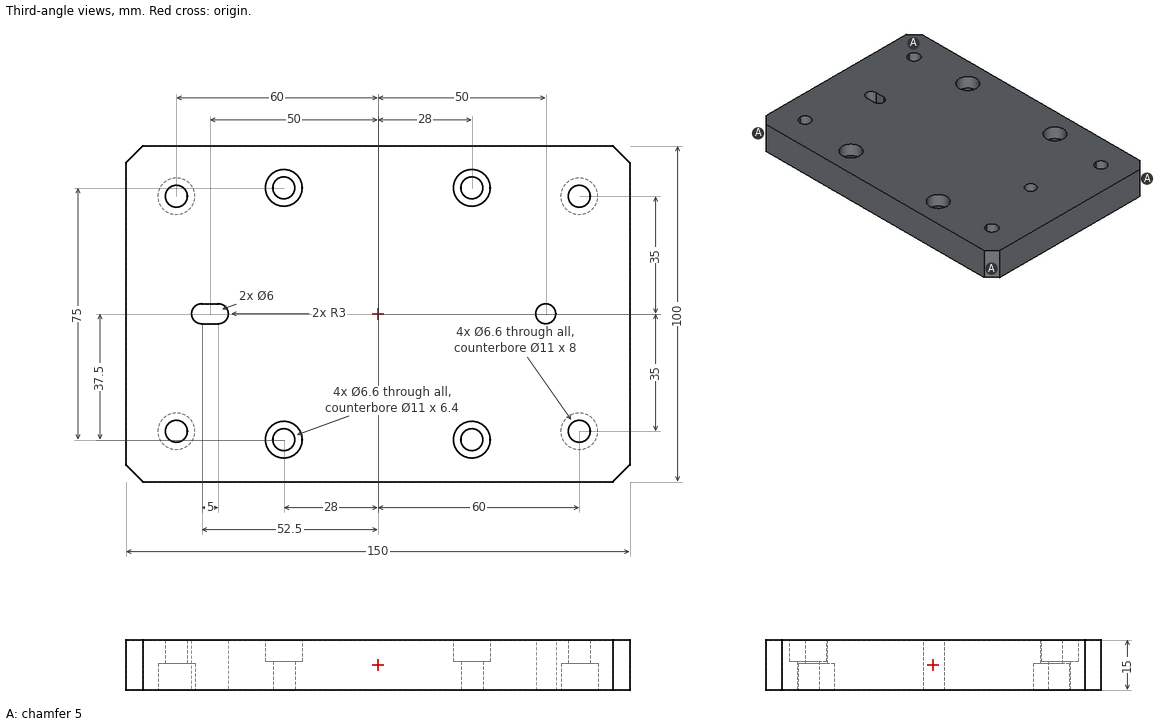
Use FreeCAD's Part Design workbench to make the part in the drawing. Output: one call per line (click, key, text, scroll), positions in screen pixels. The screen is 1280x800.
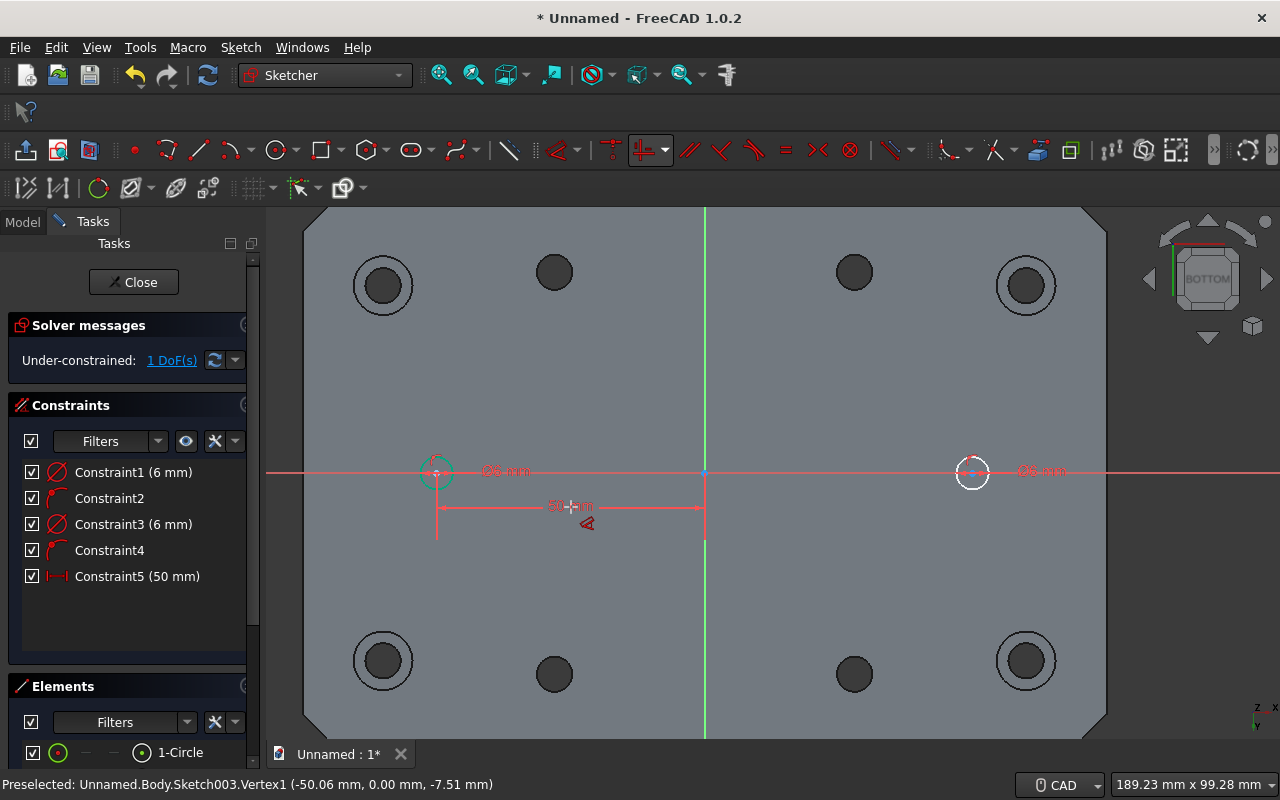
click(973, 473)
click(839, 507)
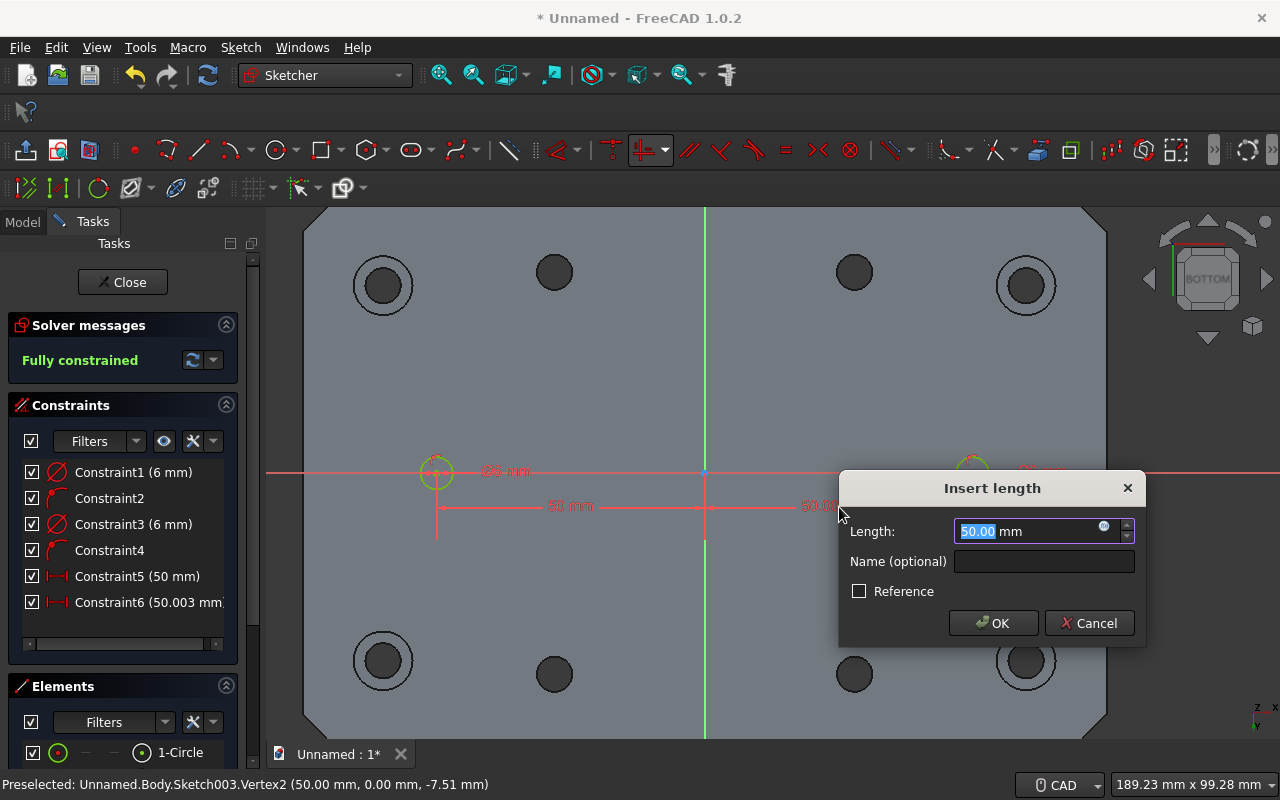
text(50)
key(Return)
key(Escape)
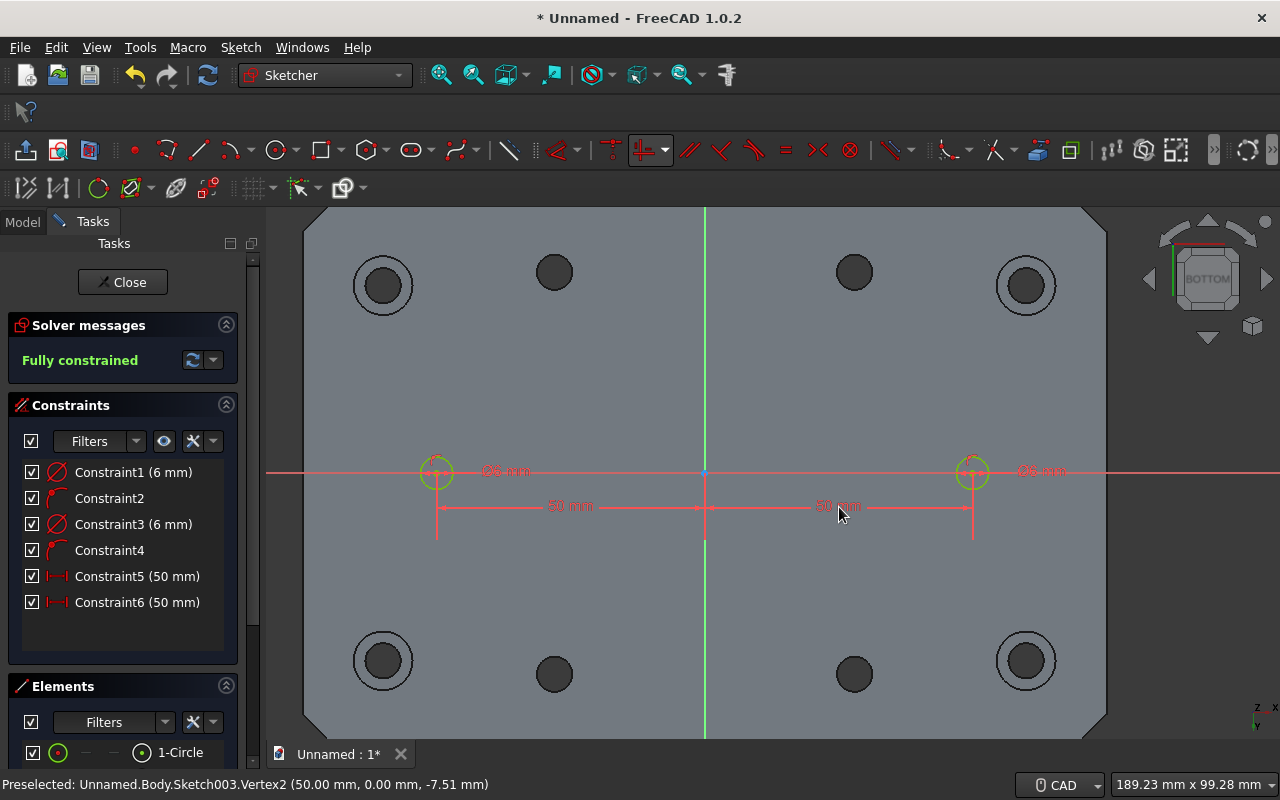
click(123, 282)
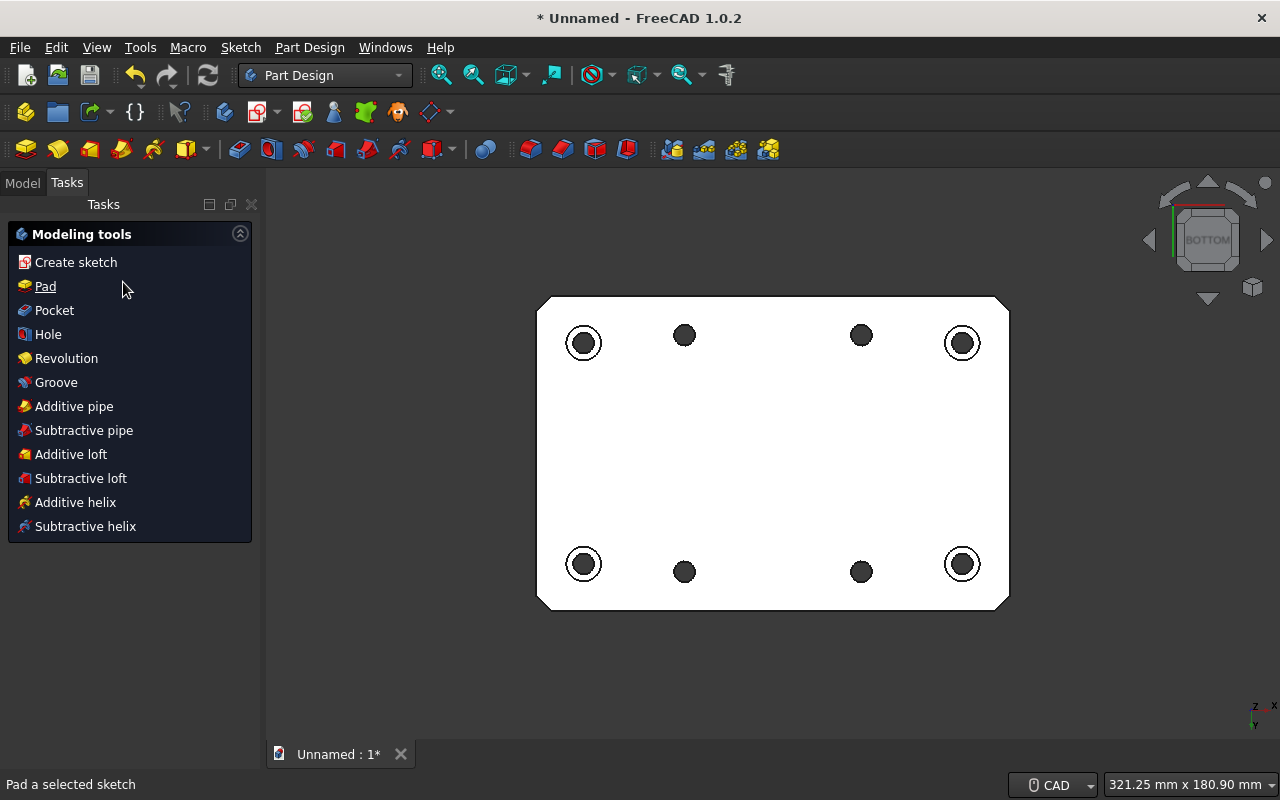
click(240, 150)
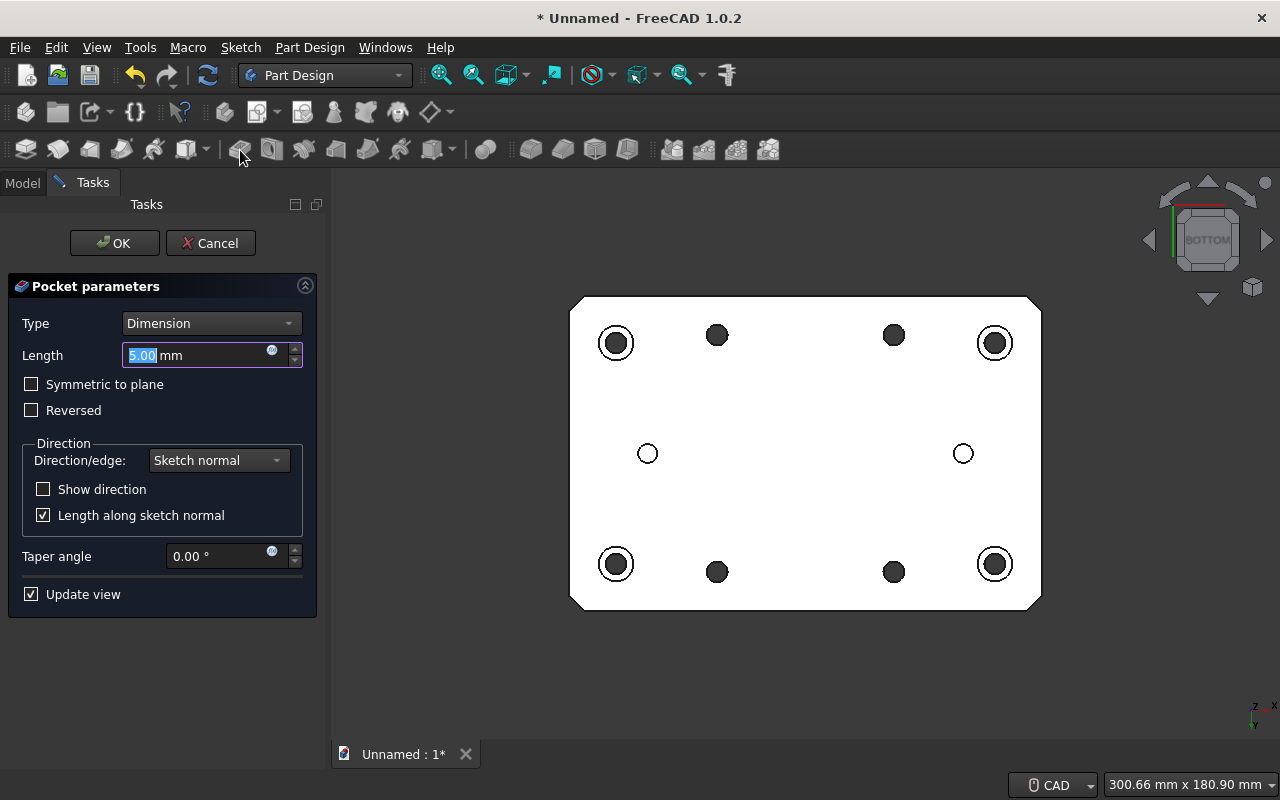
click(212, 324)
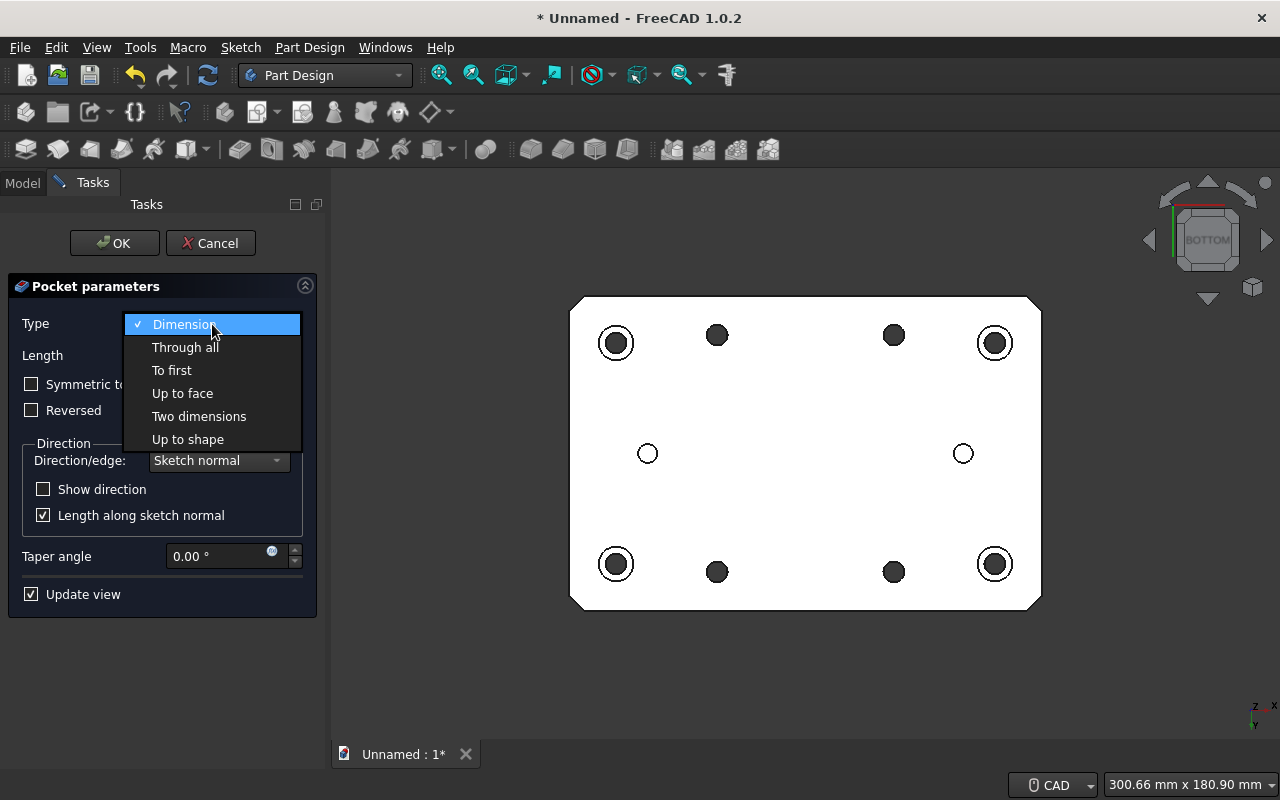
click(212, 348)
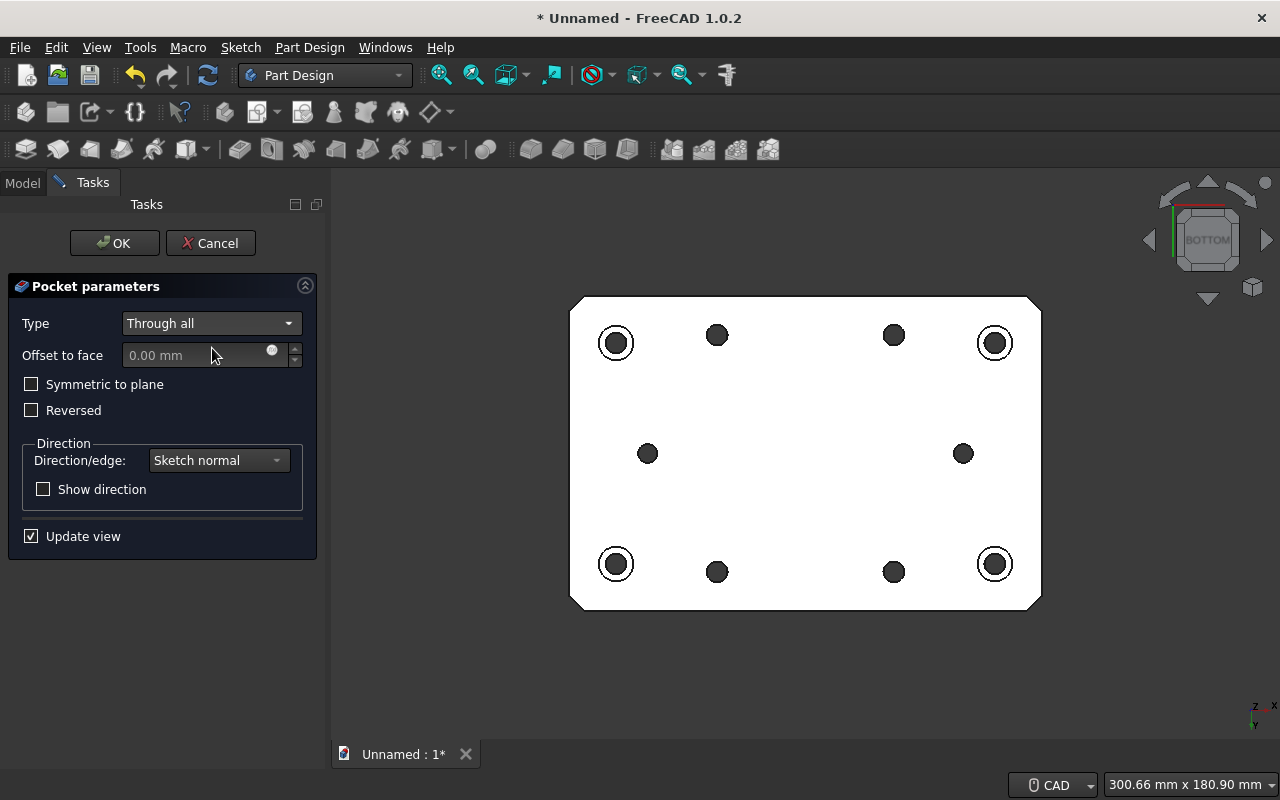
click(115, 243)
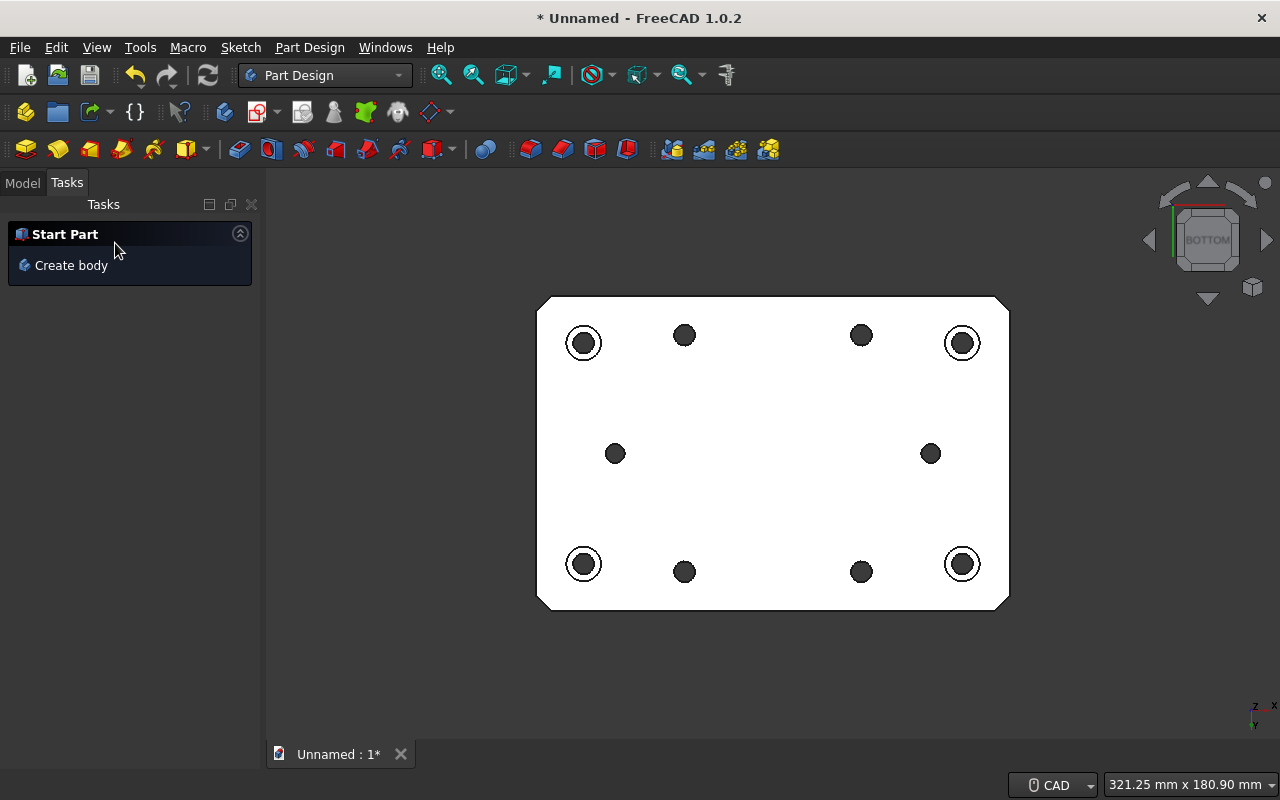
click(773, 453)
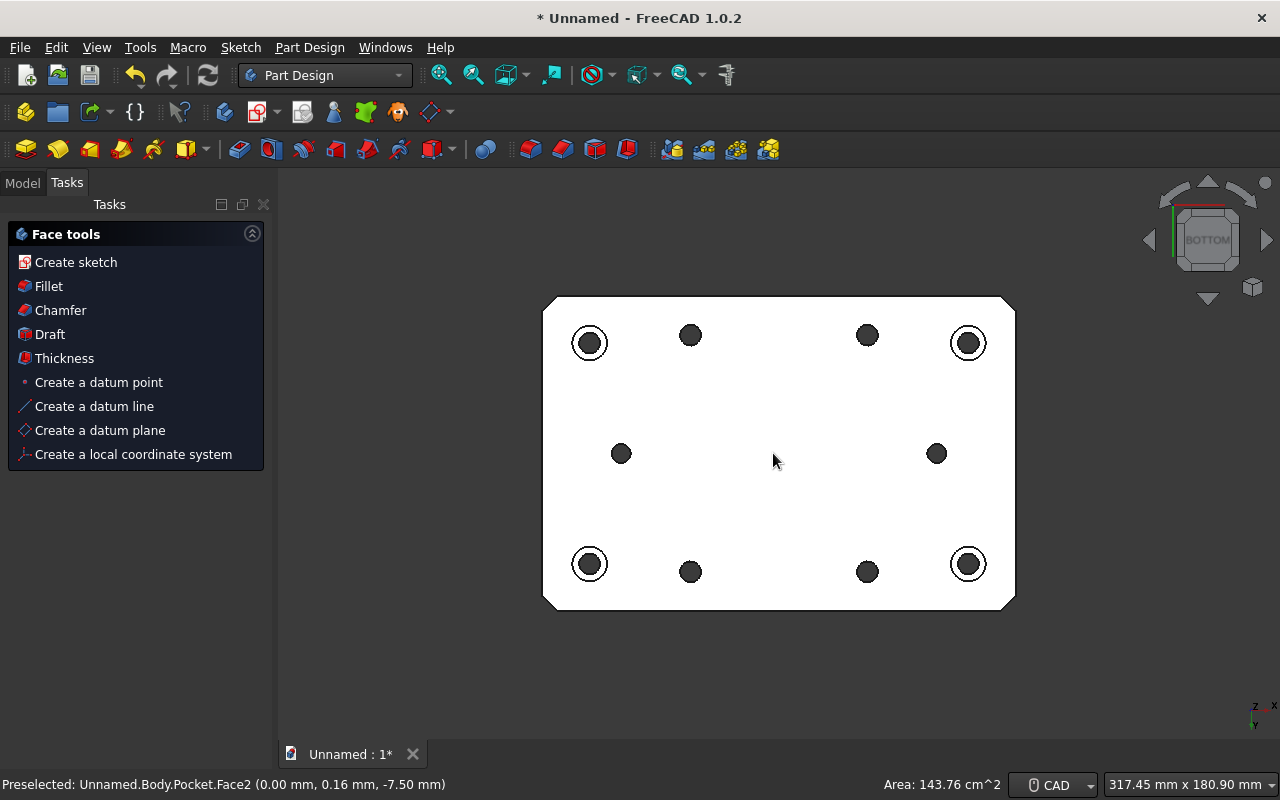
click(258, 112)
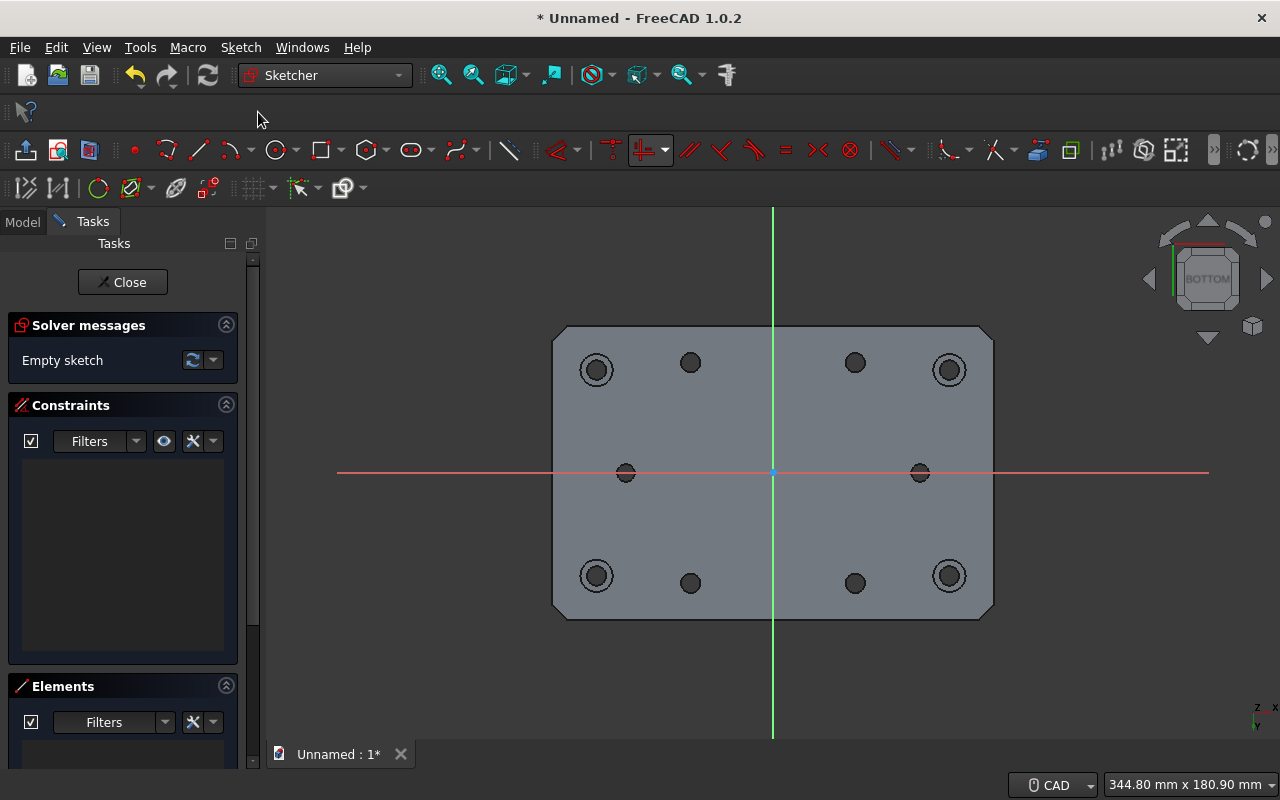
scroll(621, 473, up, 14)